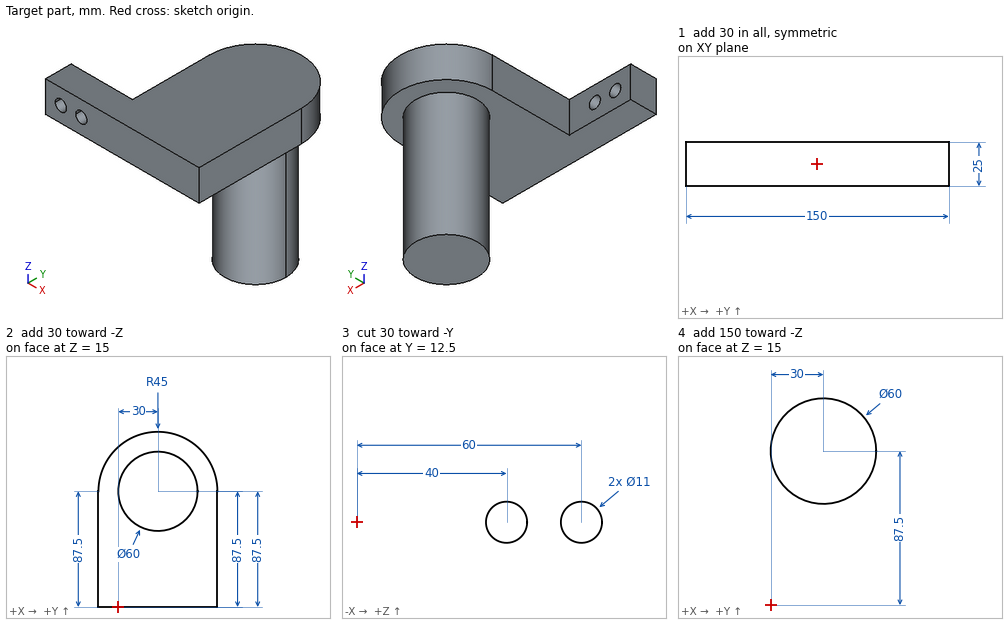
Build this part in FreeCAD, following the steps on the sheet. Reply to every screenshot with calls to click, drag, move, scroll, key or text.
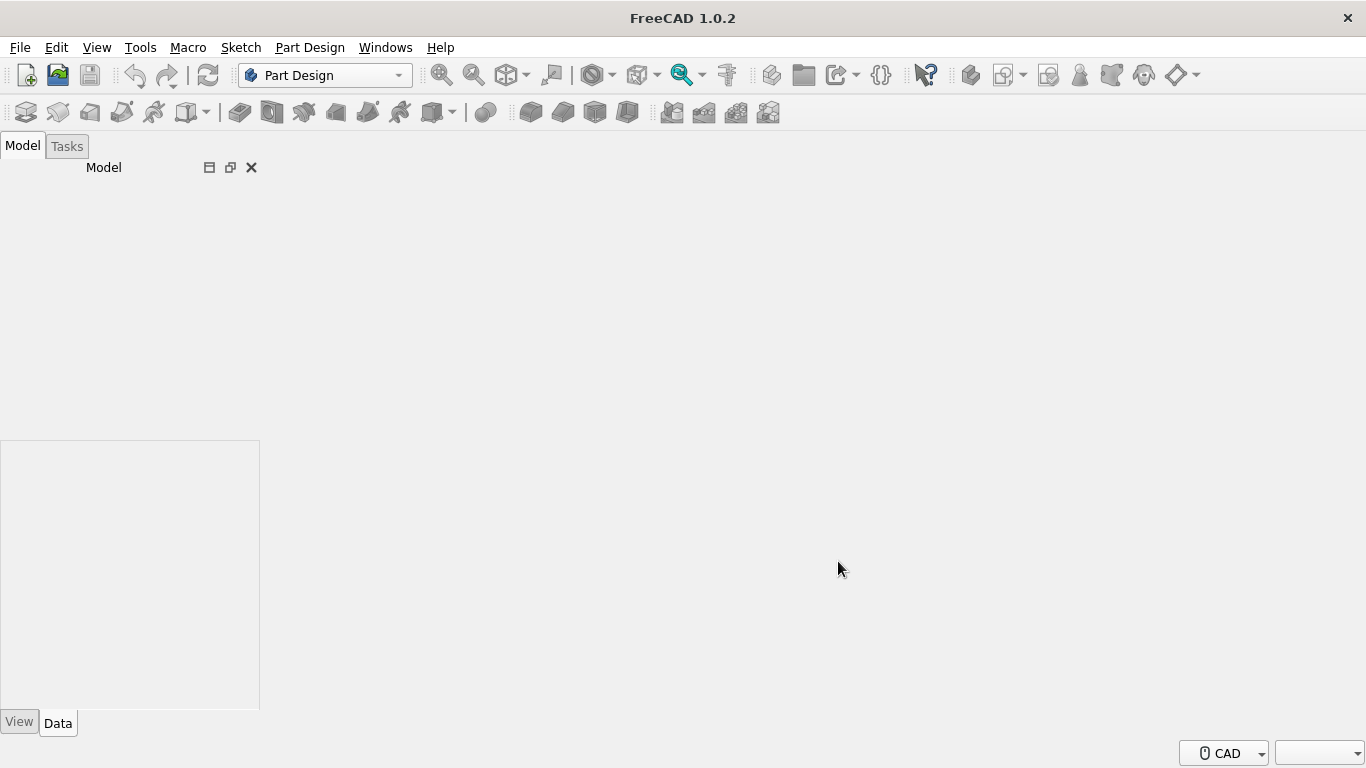
click(26, 76)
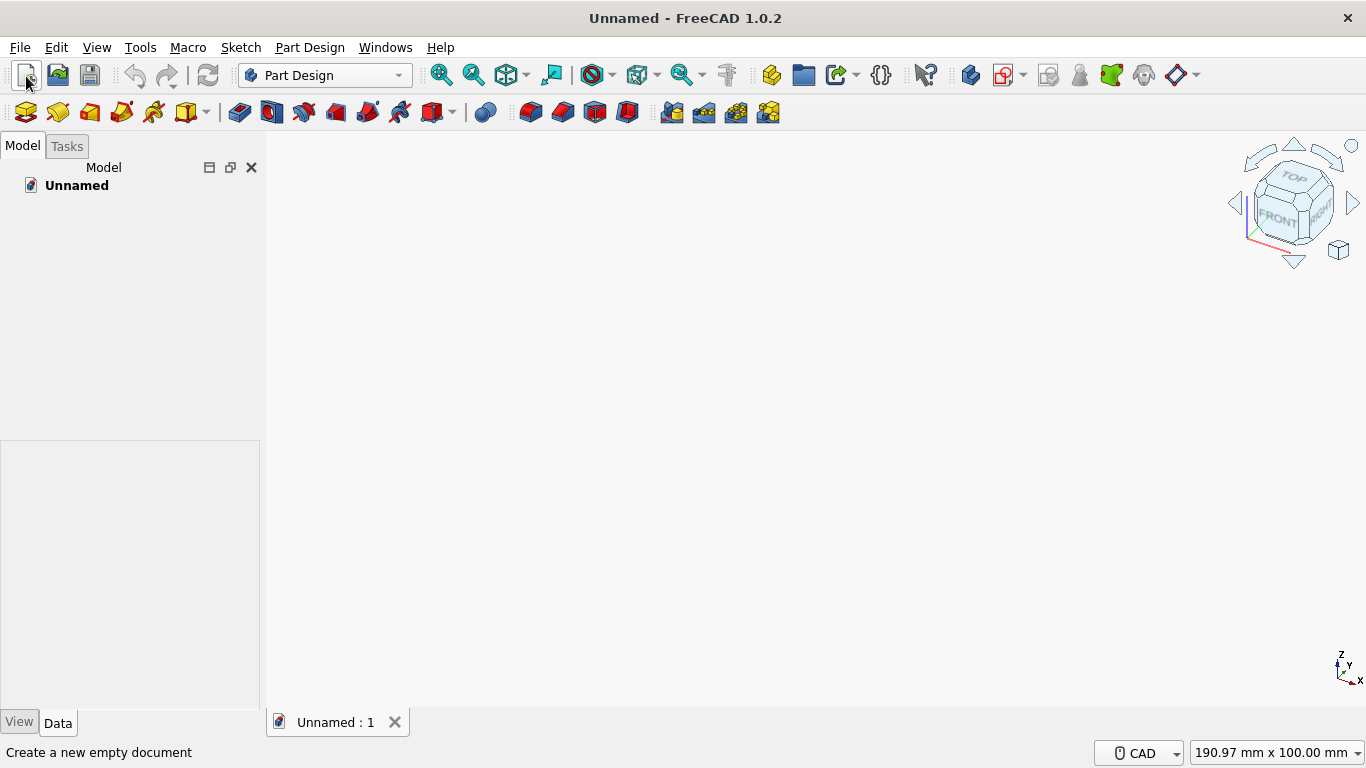
click(1004, 76)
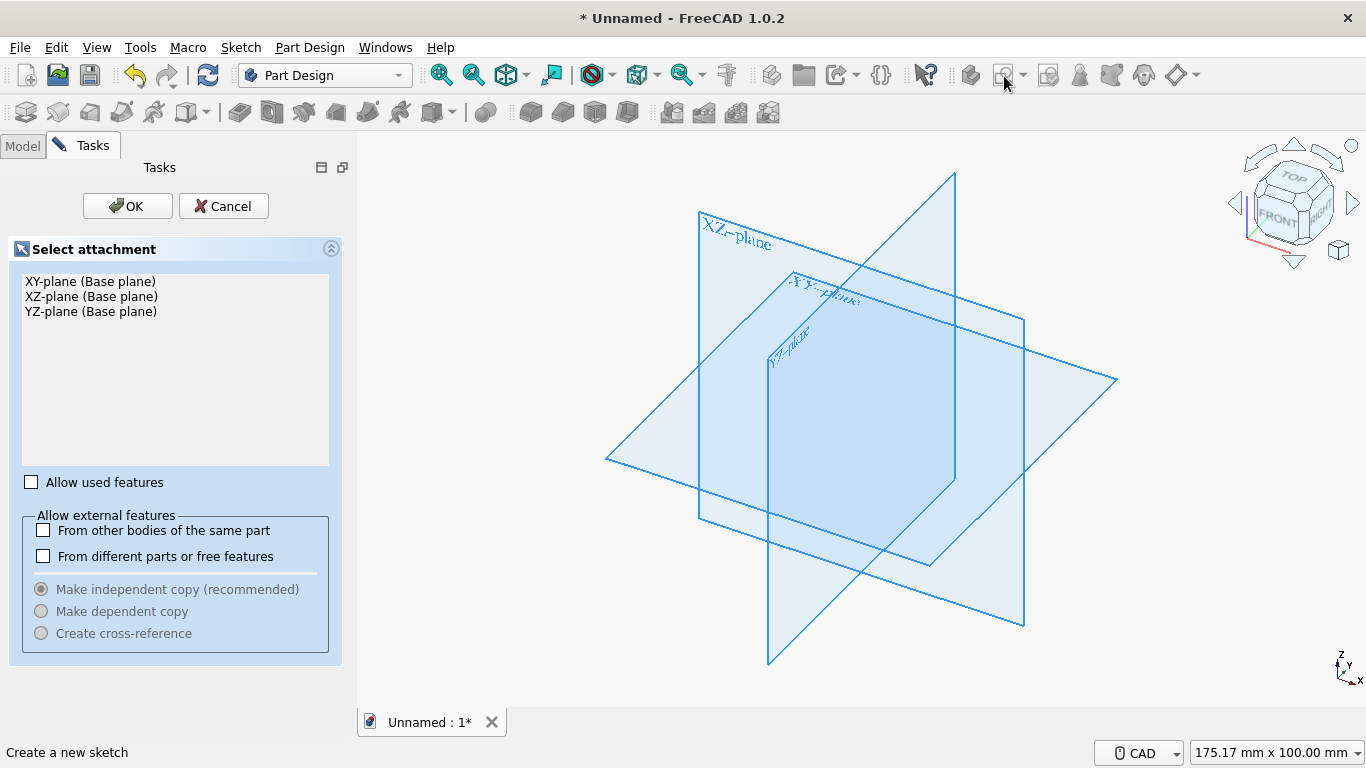
click(82, 282)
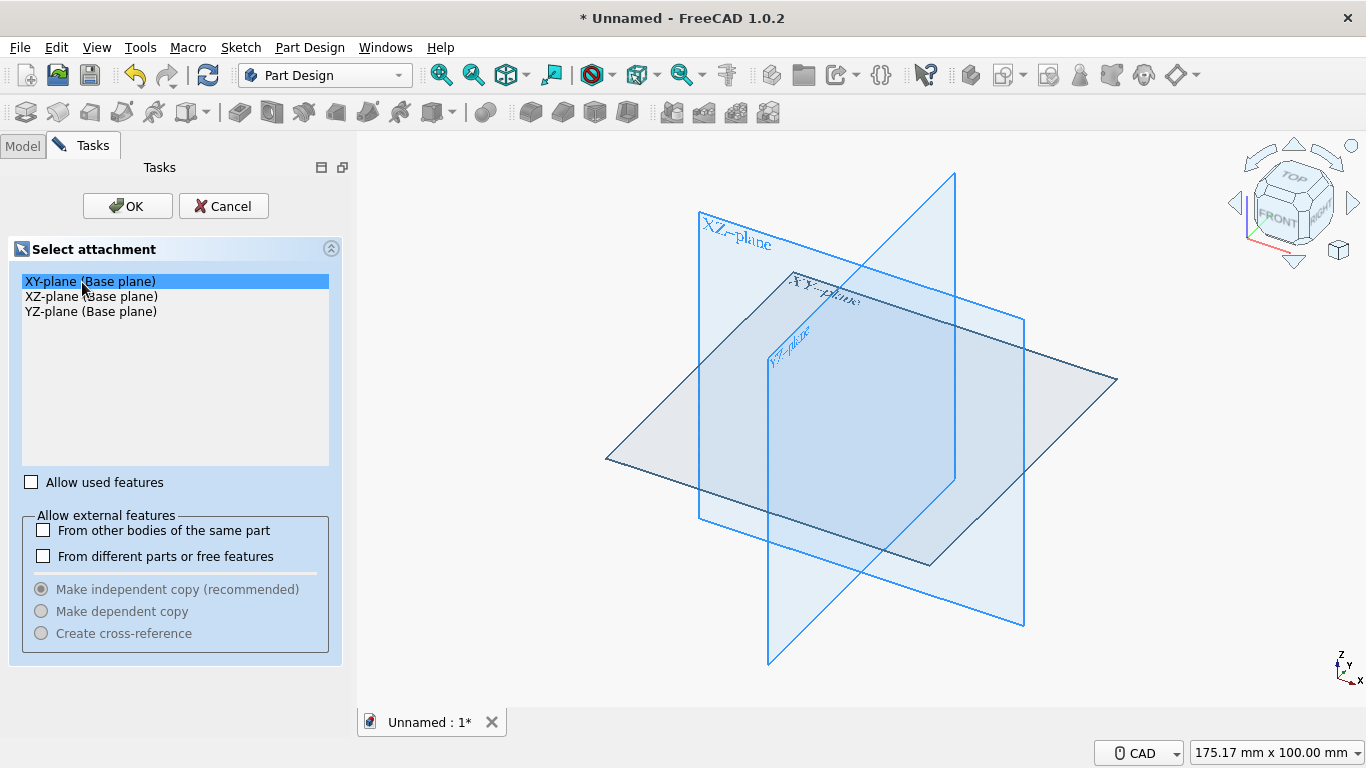
click(128, 206)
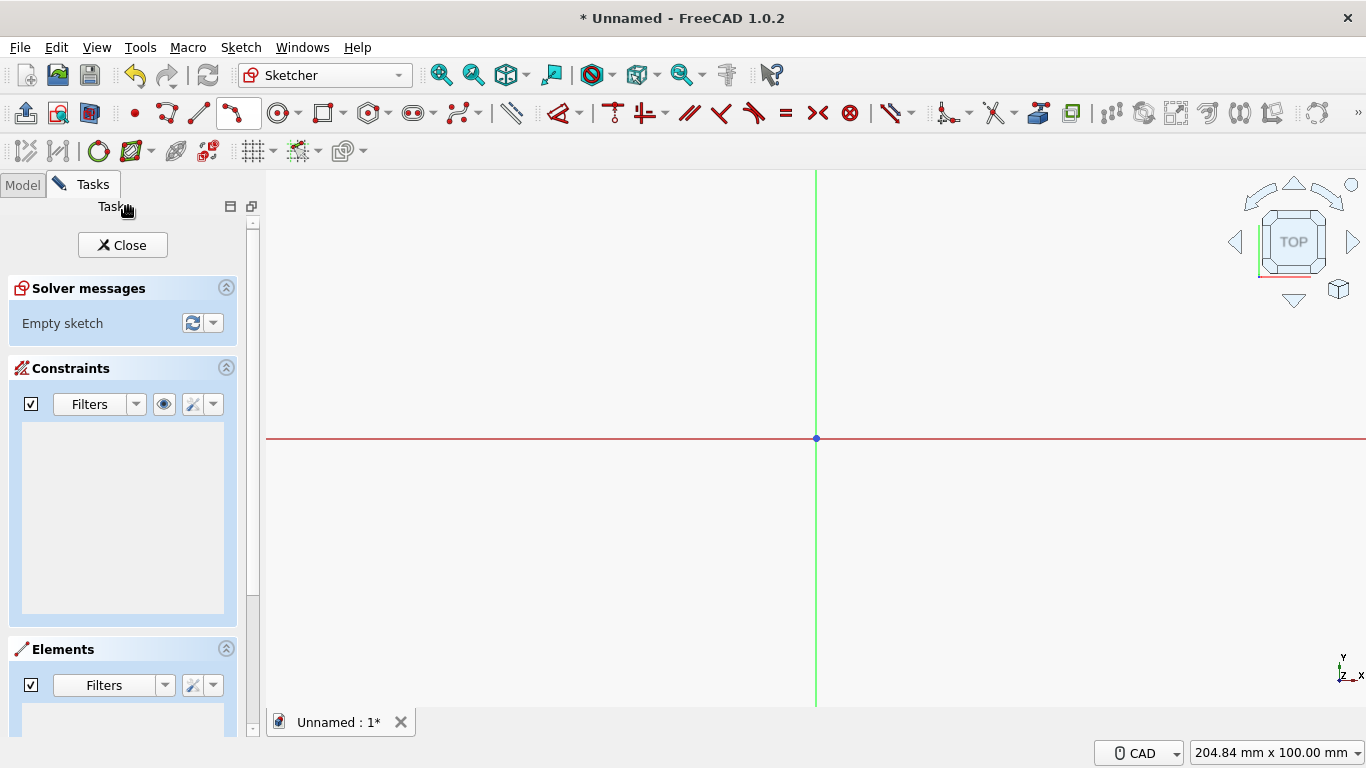
scroll(438, 439, down, 1)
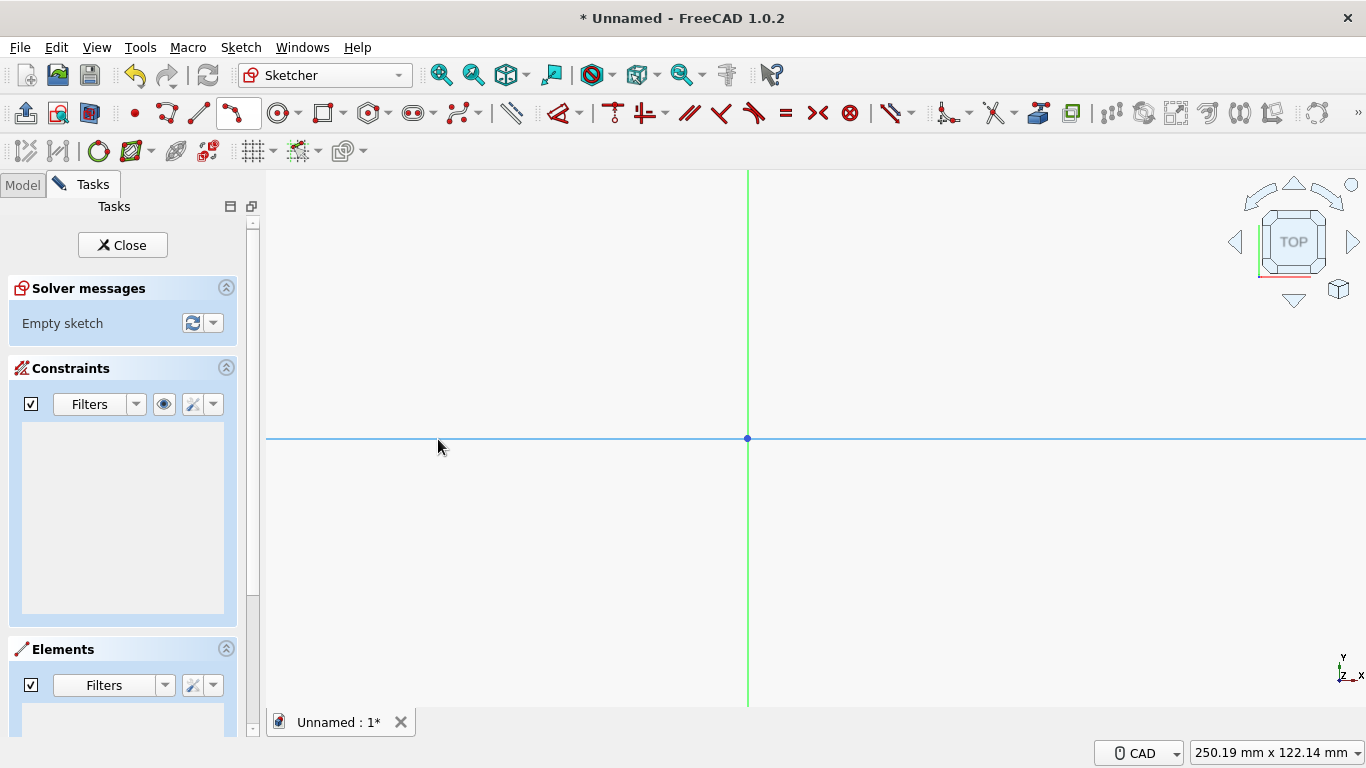
click(346, 114)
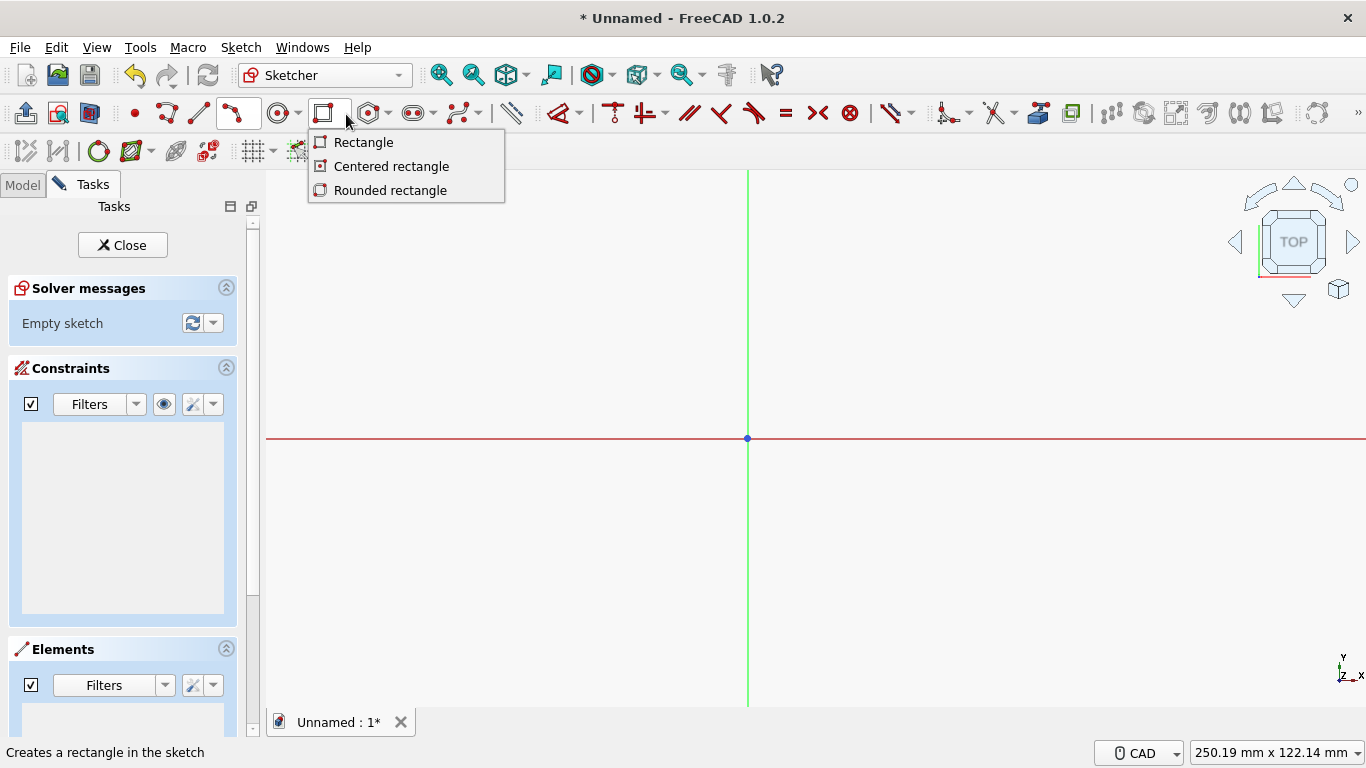
click(406, 166)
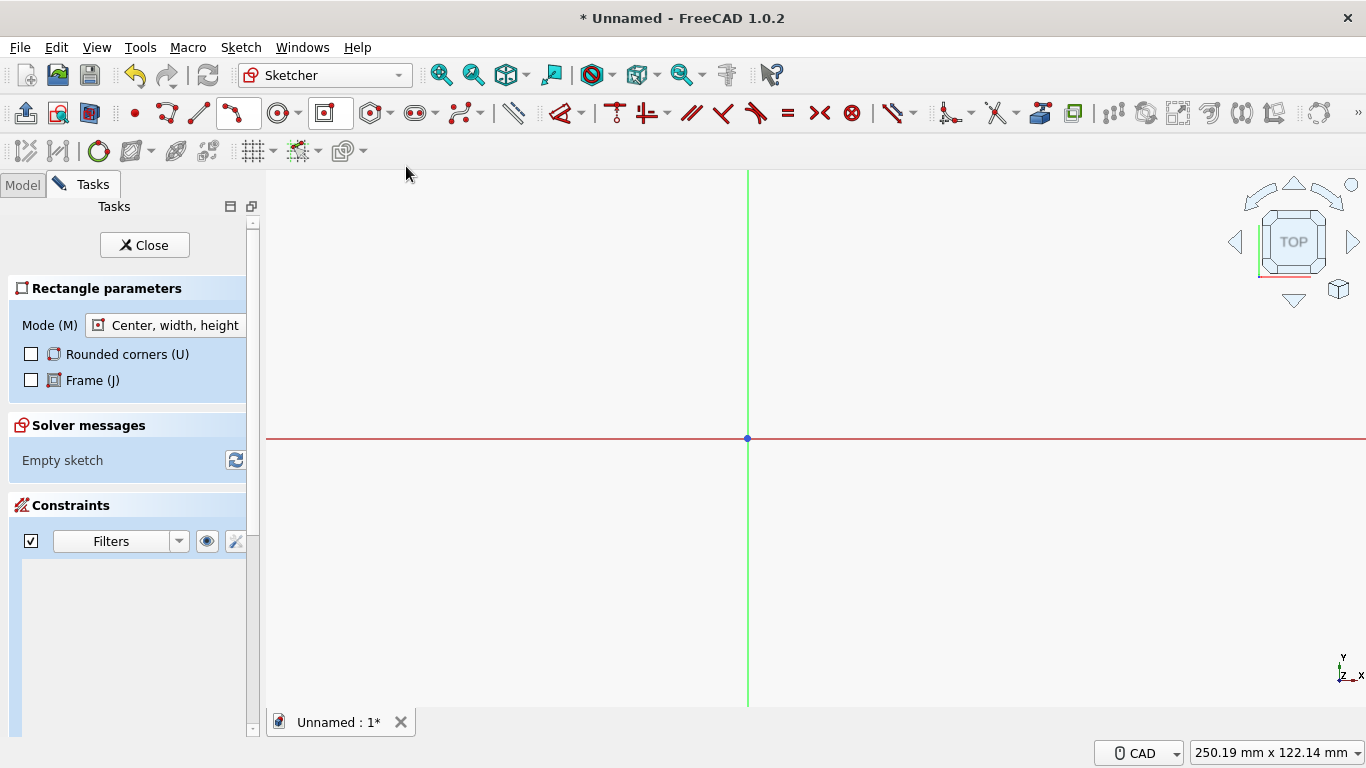
click(748, 439)
click(1077, 384)
key(Escape)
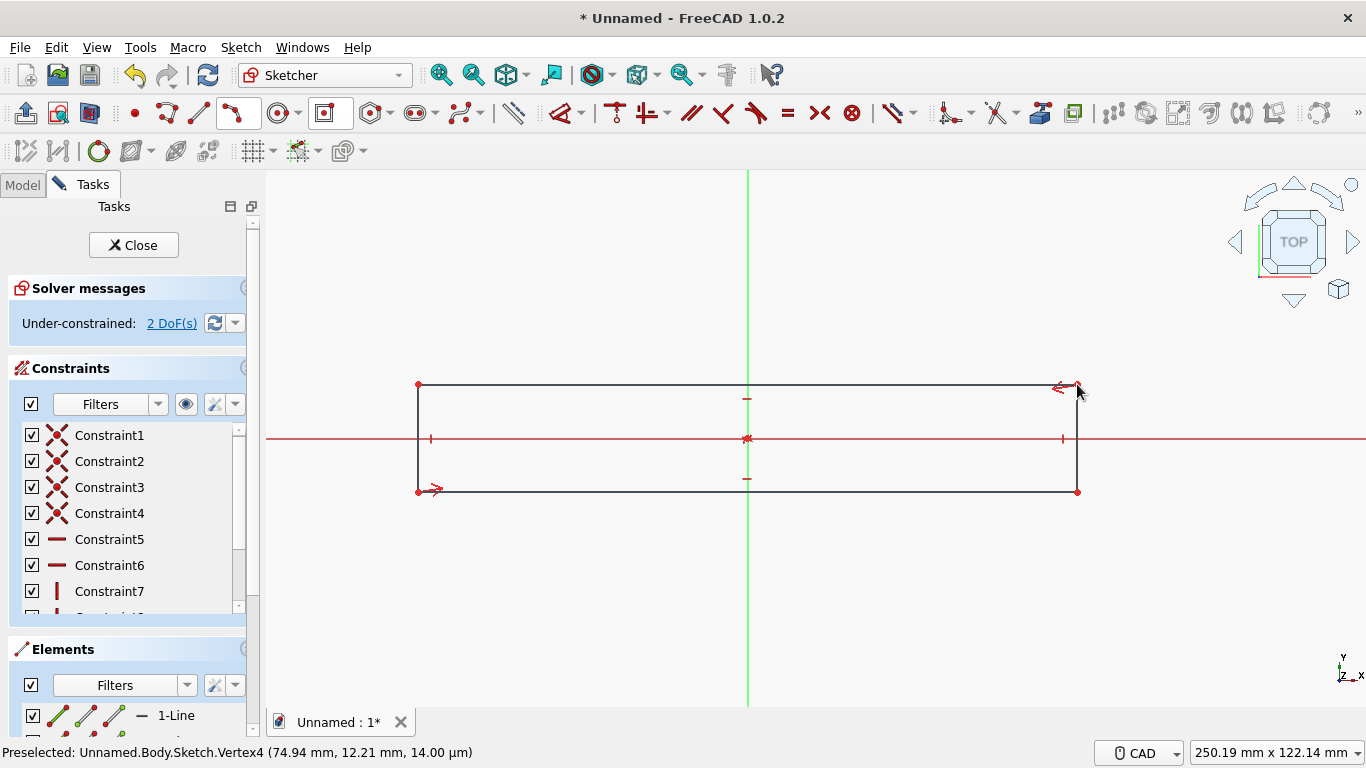
key(d)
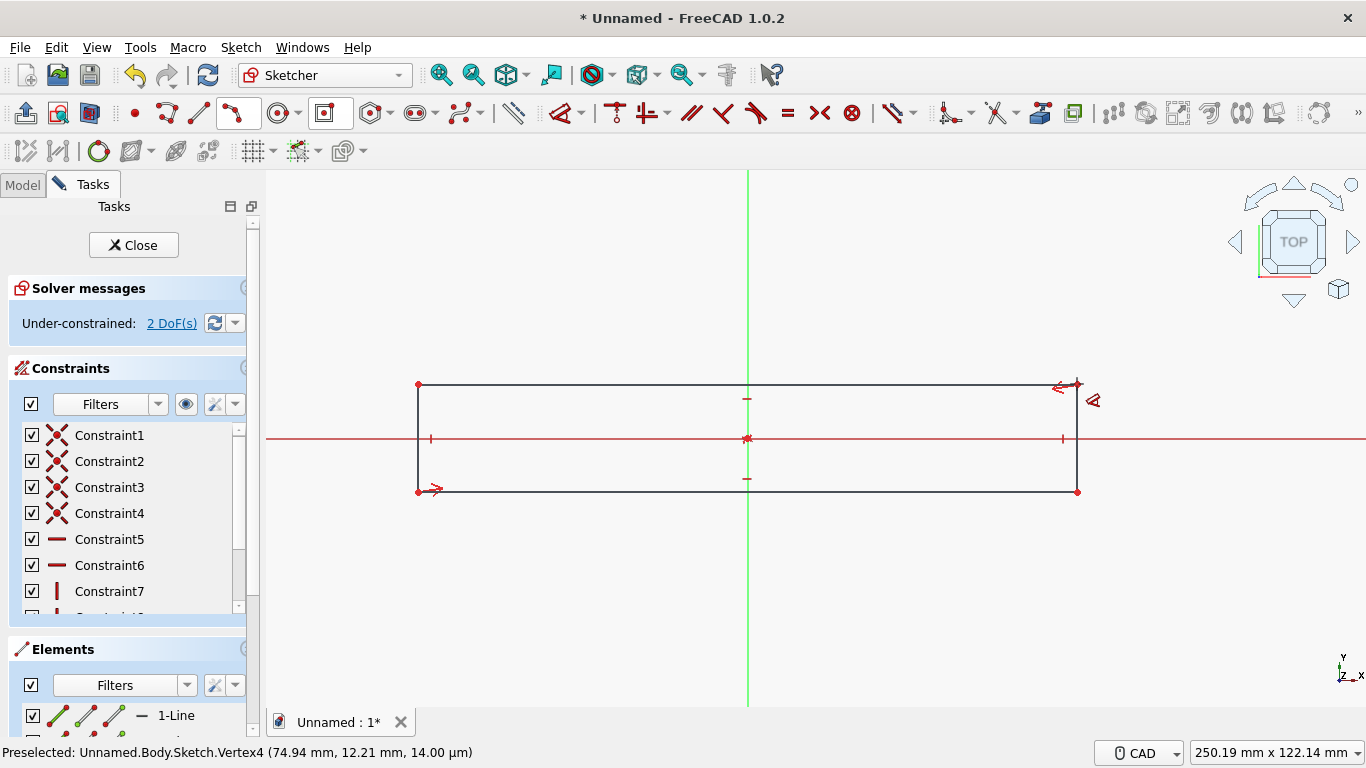
click(1077, 460)
click(1111, 414)